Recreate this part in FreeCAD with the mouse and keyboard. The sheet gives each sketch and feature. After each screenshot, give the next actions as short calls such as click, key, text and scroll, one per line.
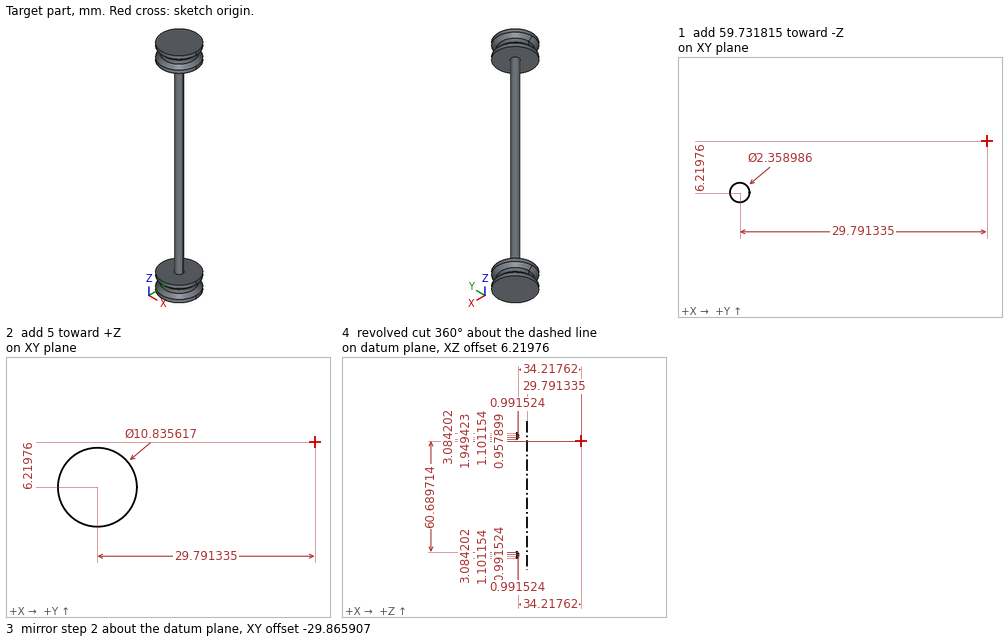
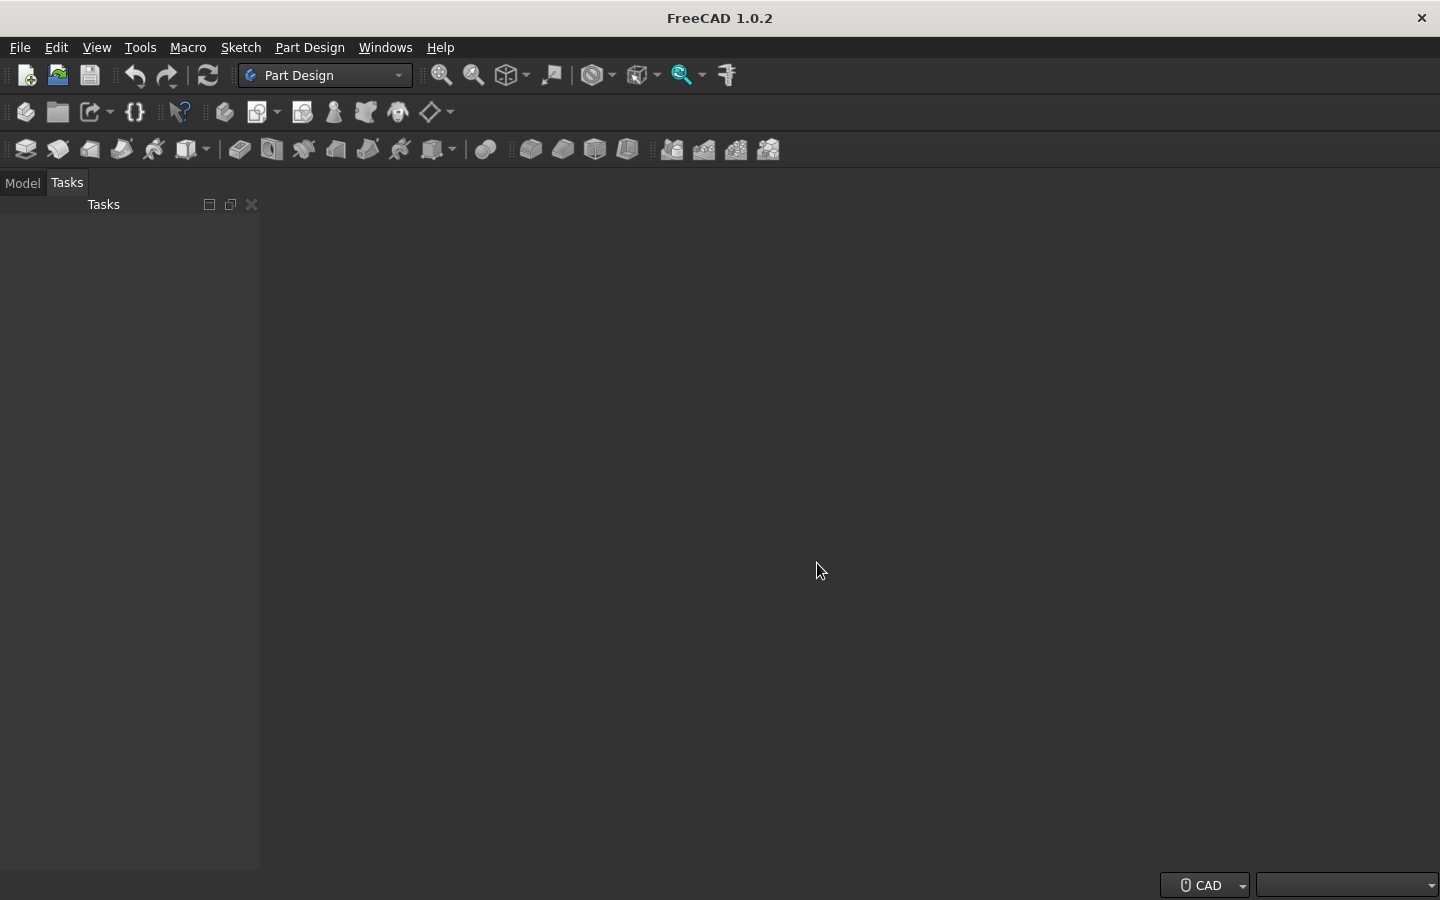
click(26, 76)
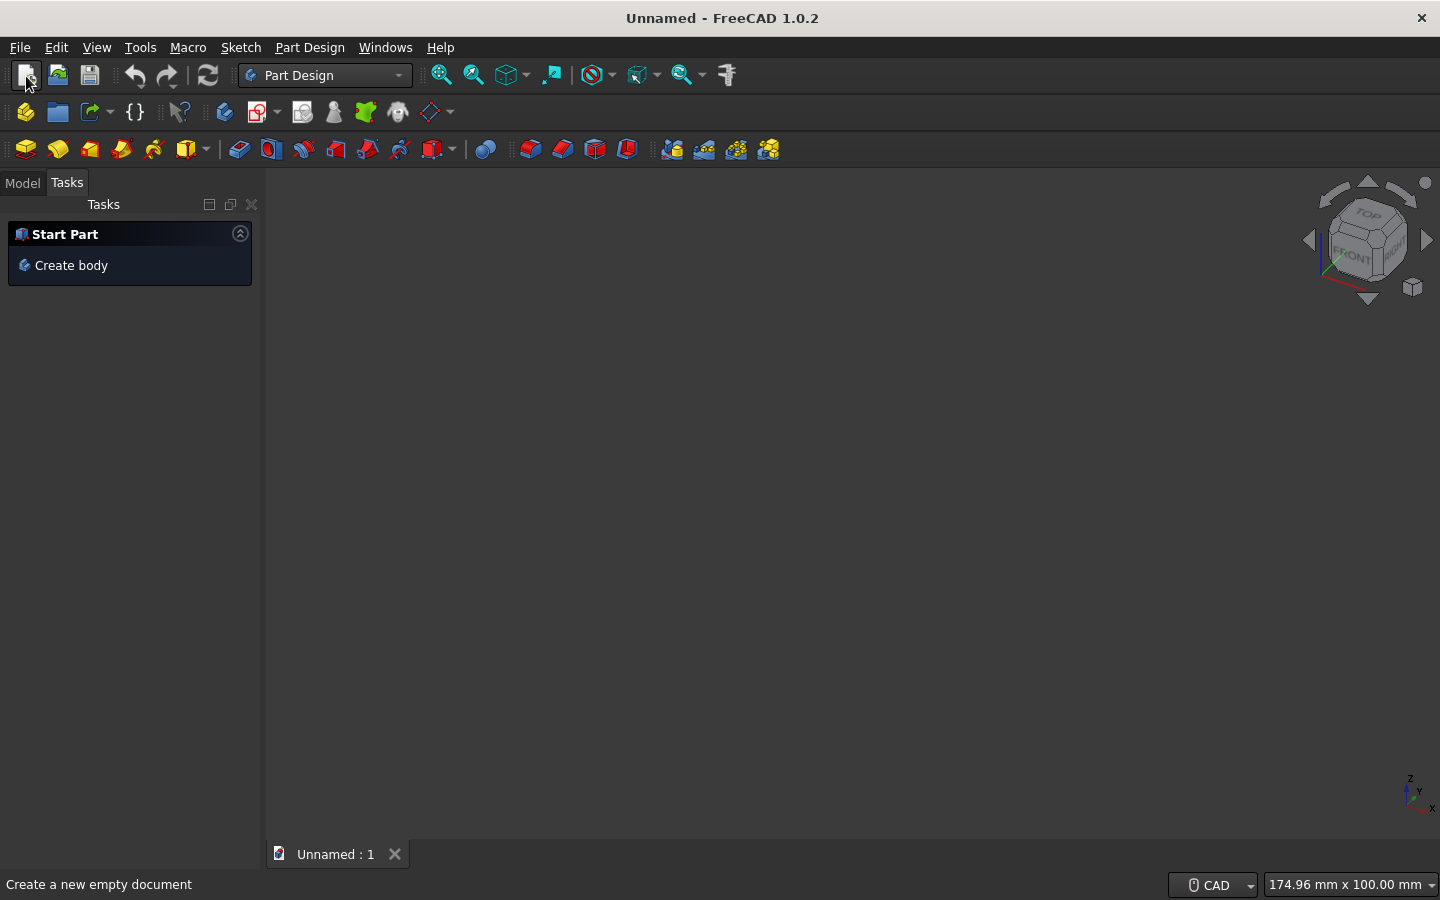
click(258, 112)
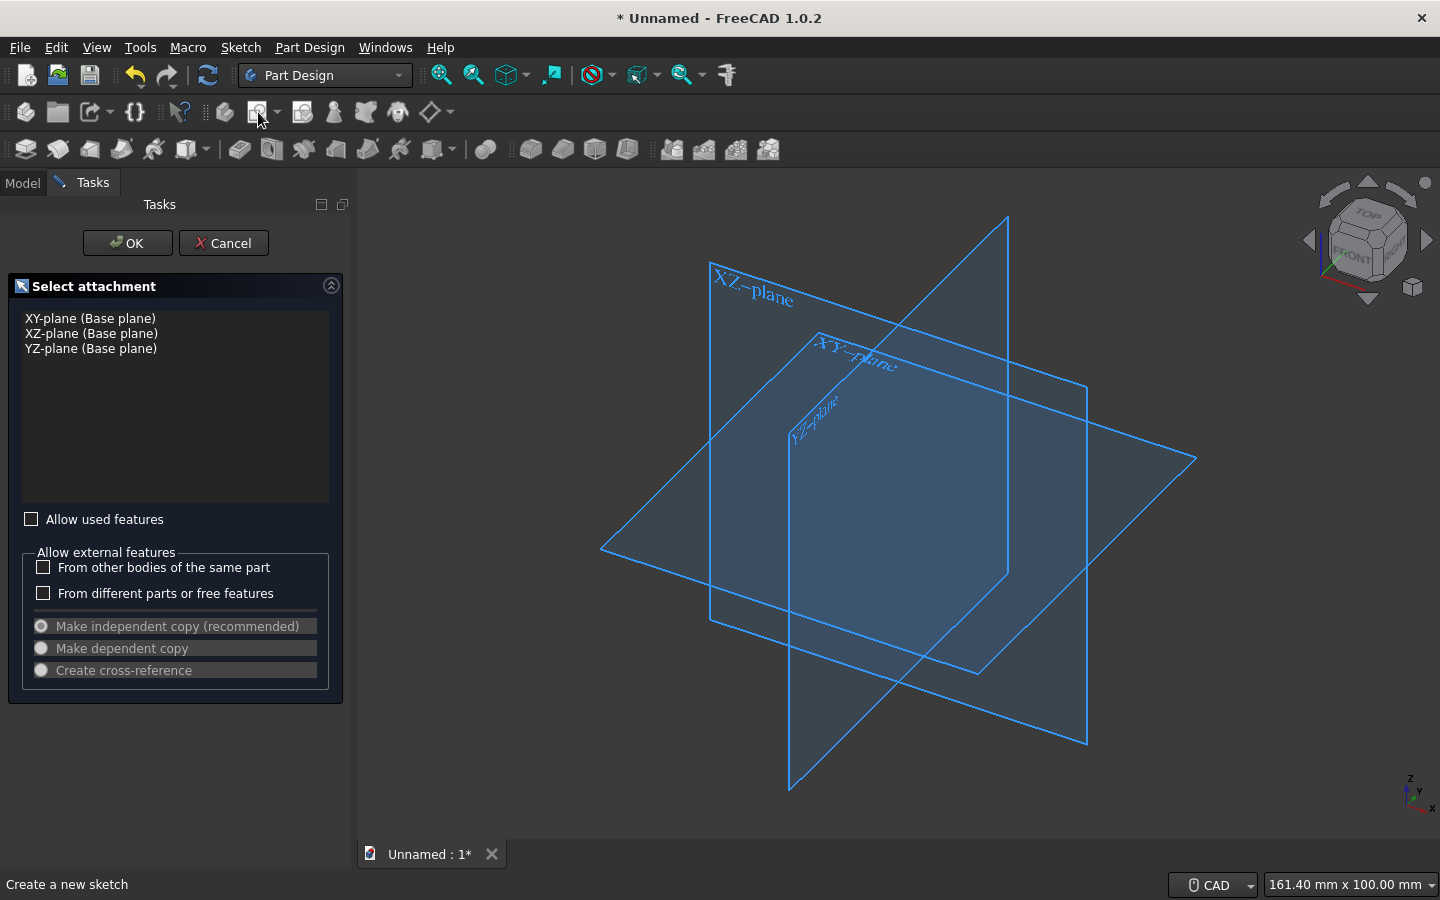
click(82, 318)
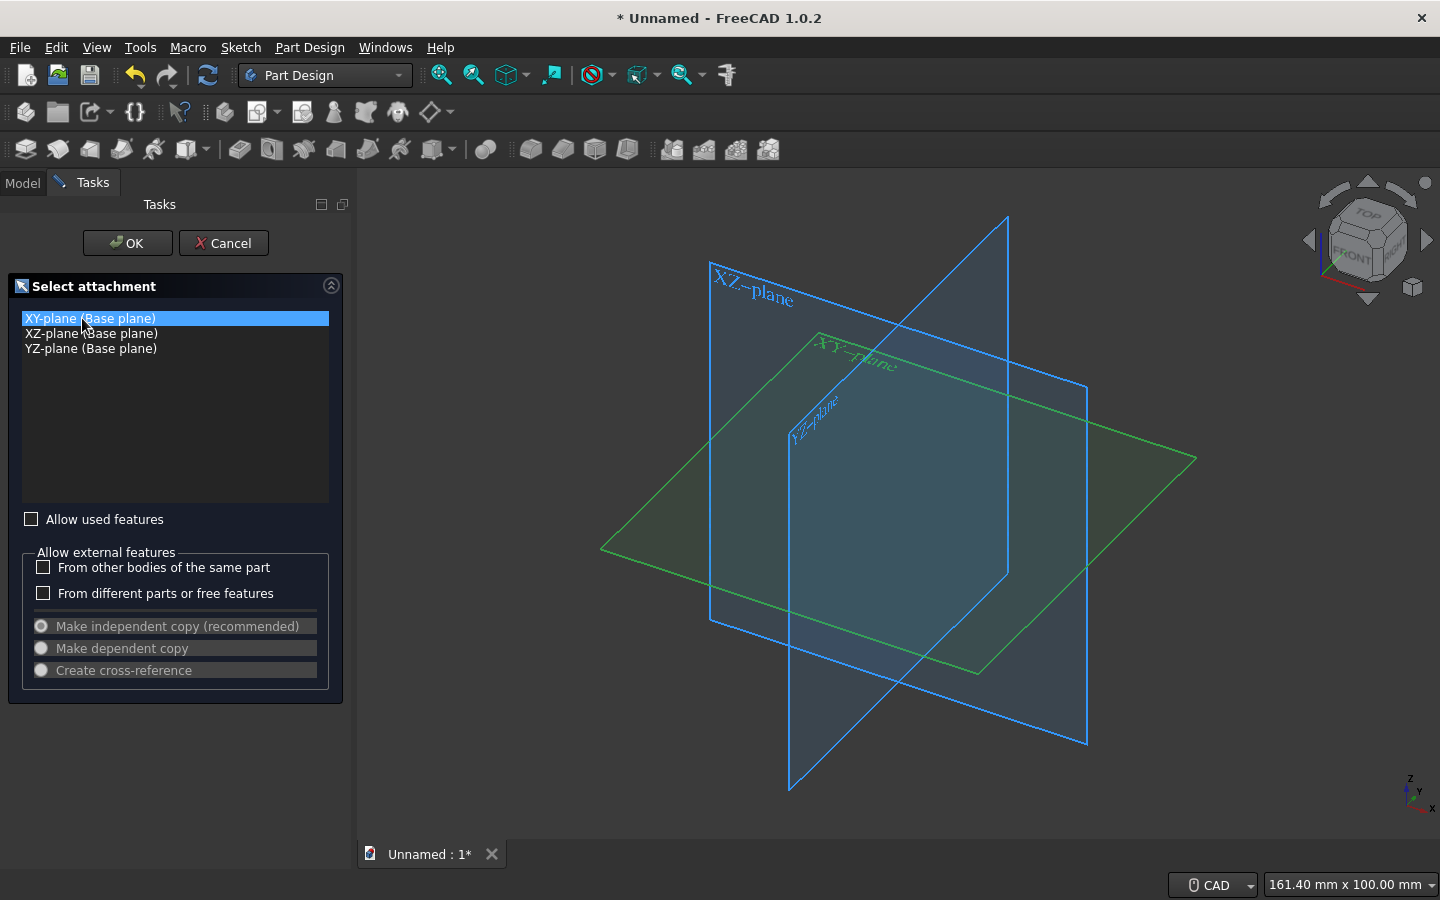
click(128, 243)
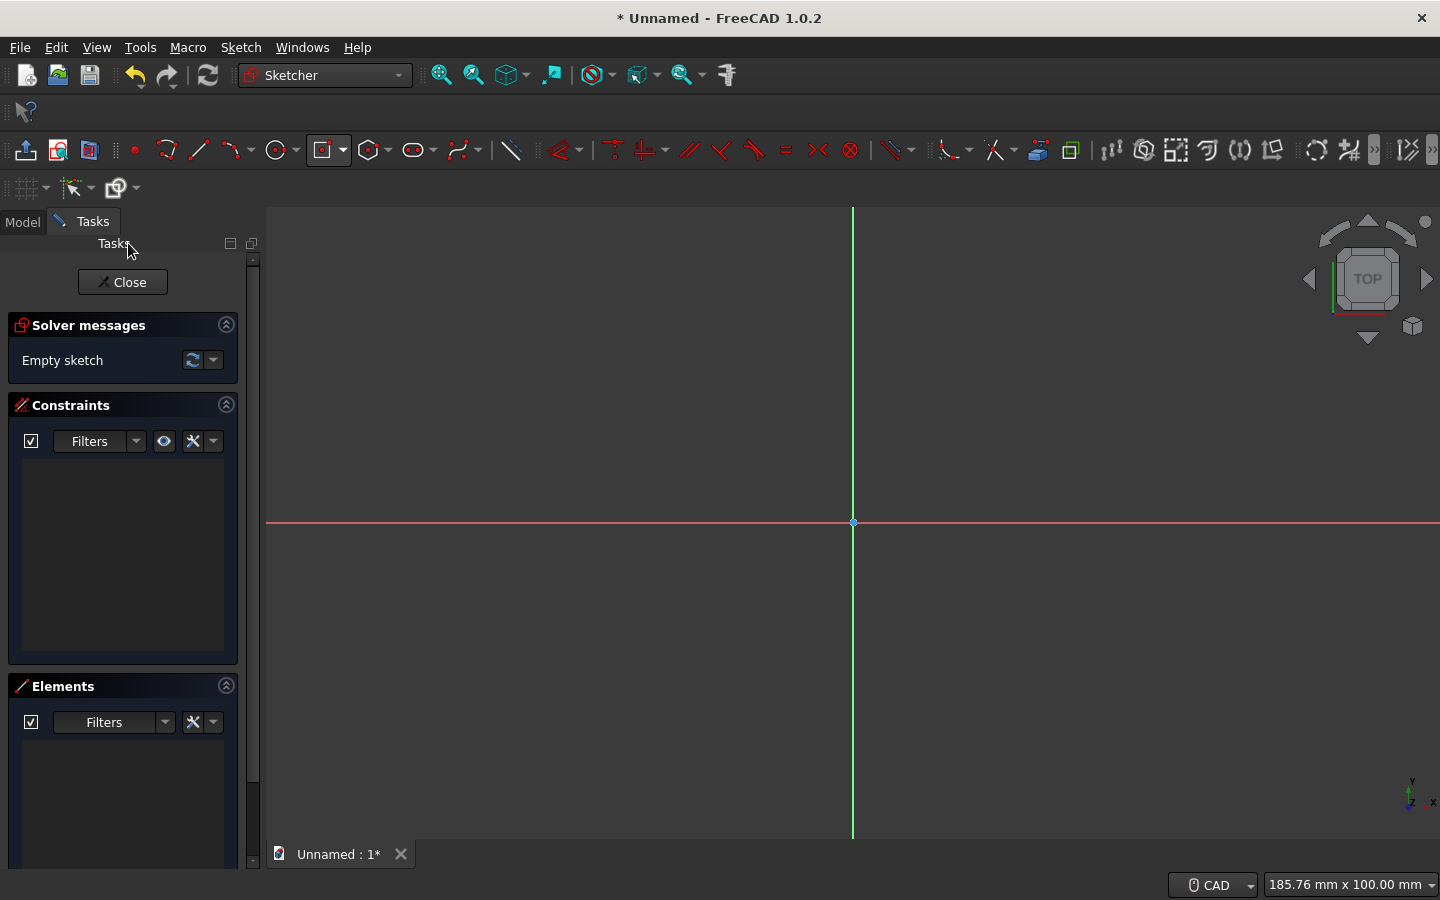
scroll(658, 564, up, 15)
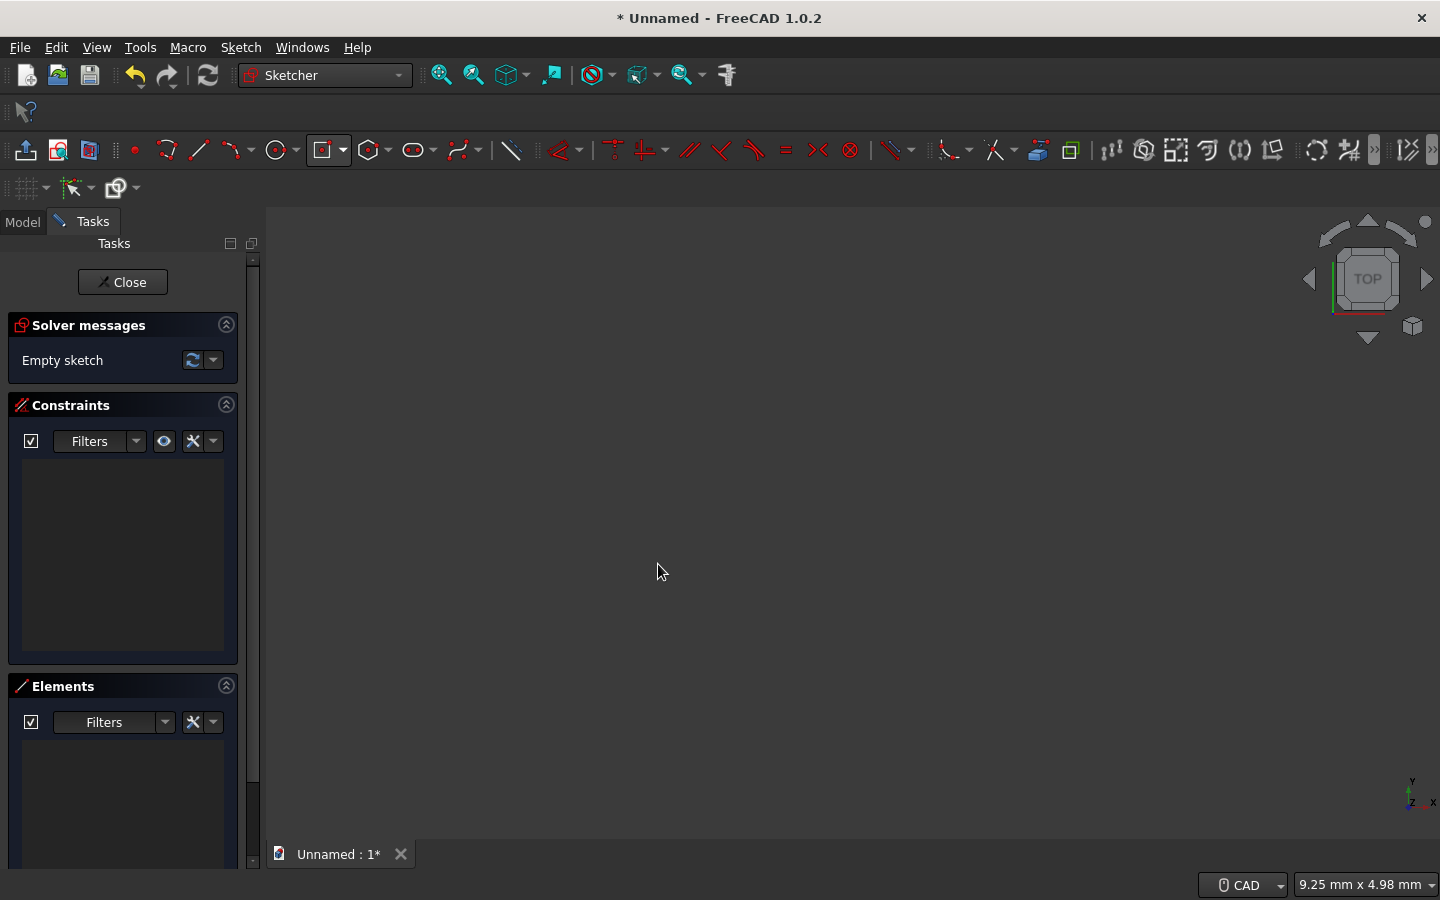
scroll(791, 512, up, 2)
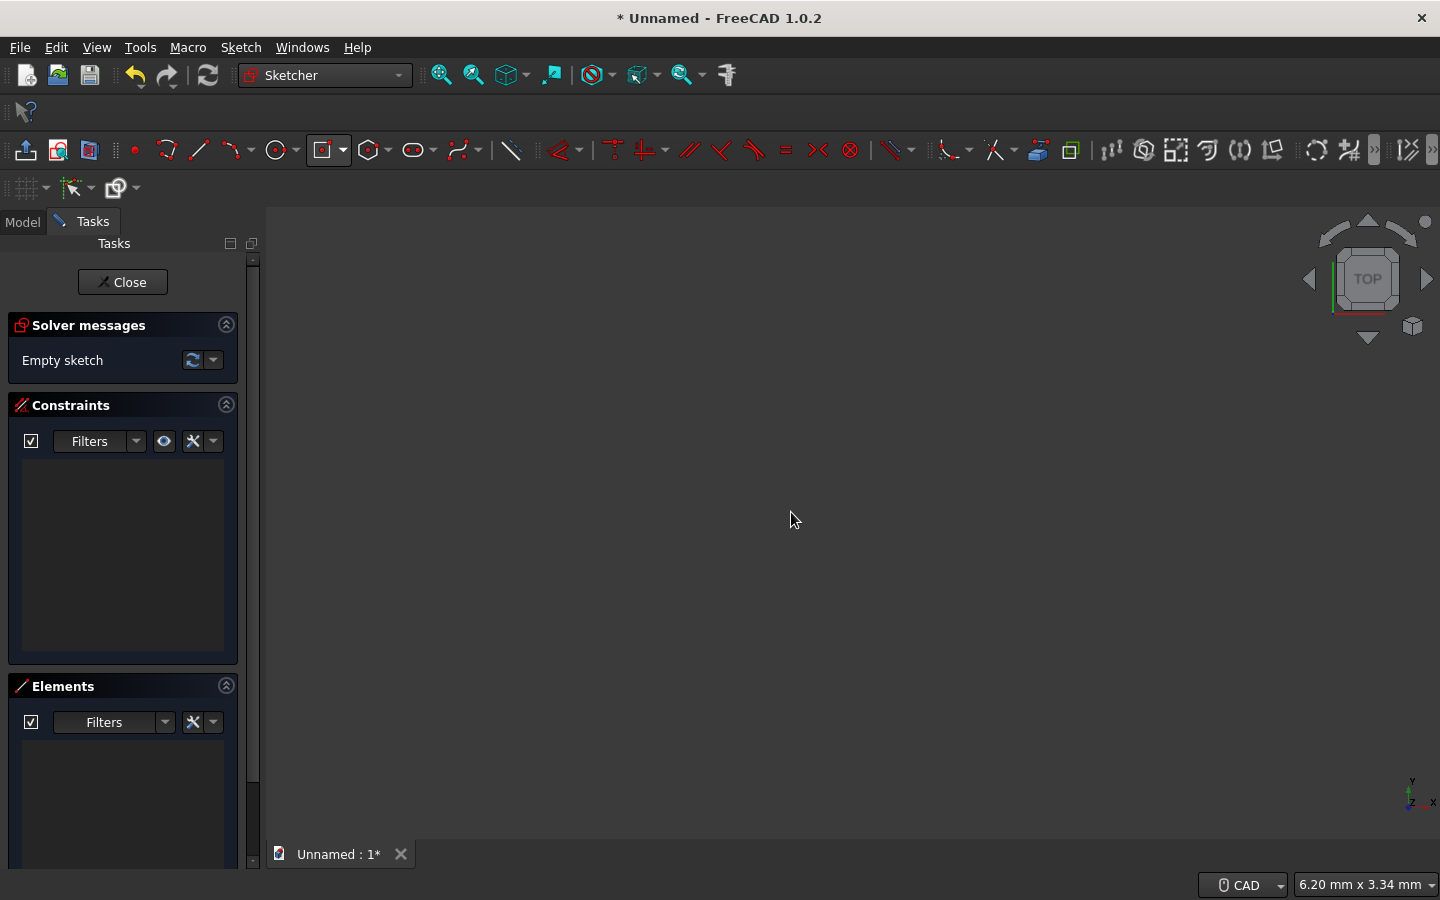
key(g)
key(c)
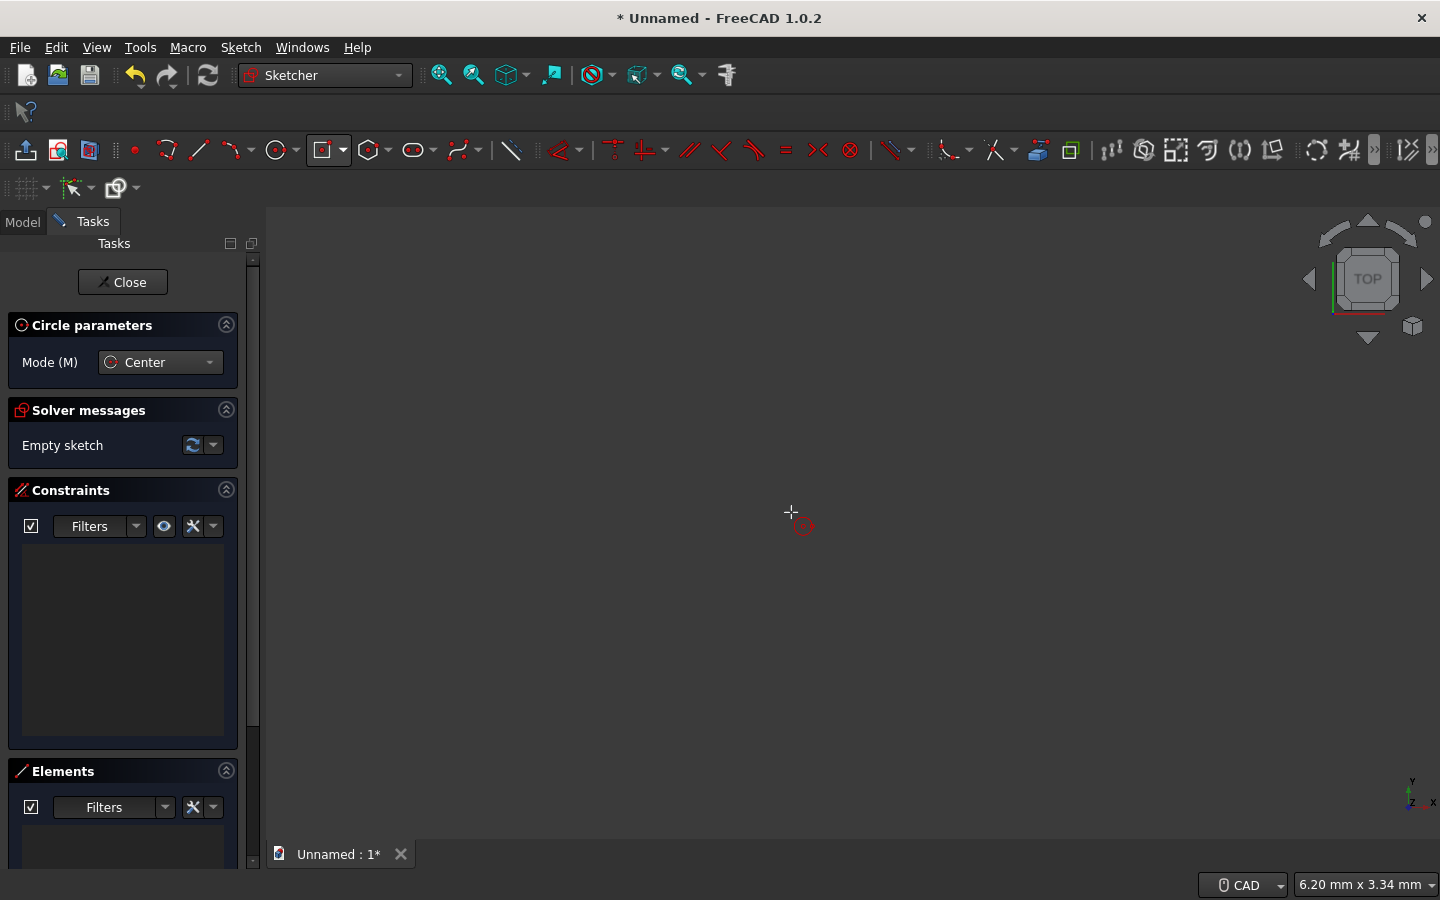
click(784, 523)
click(942, 365)
key(Escape)